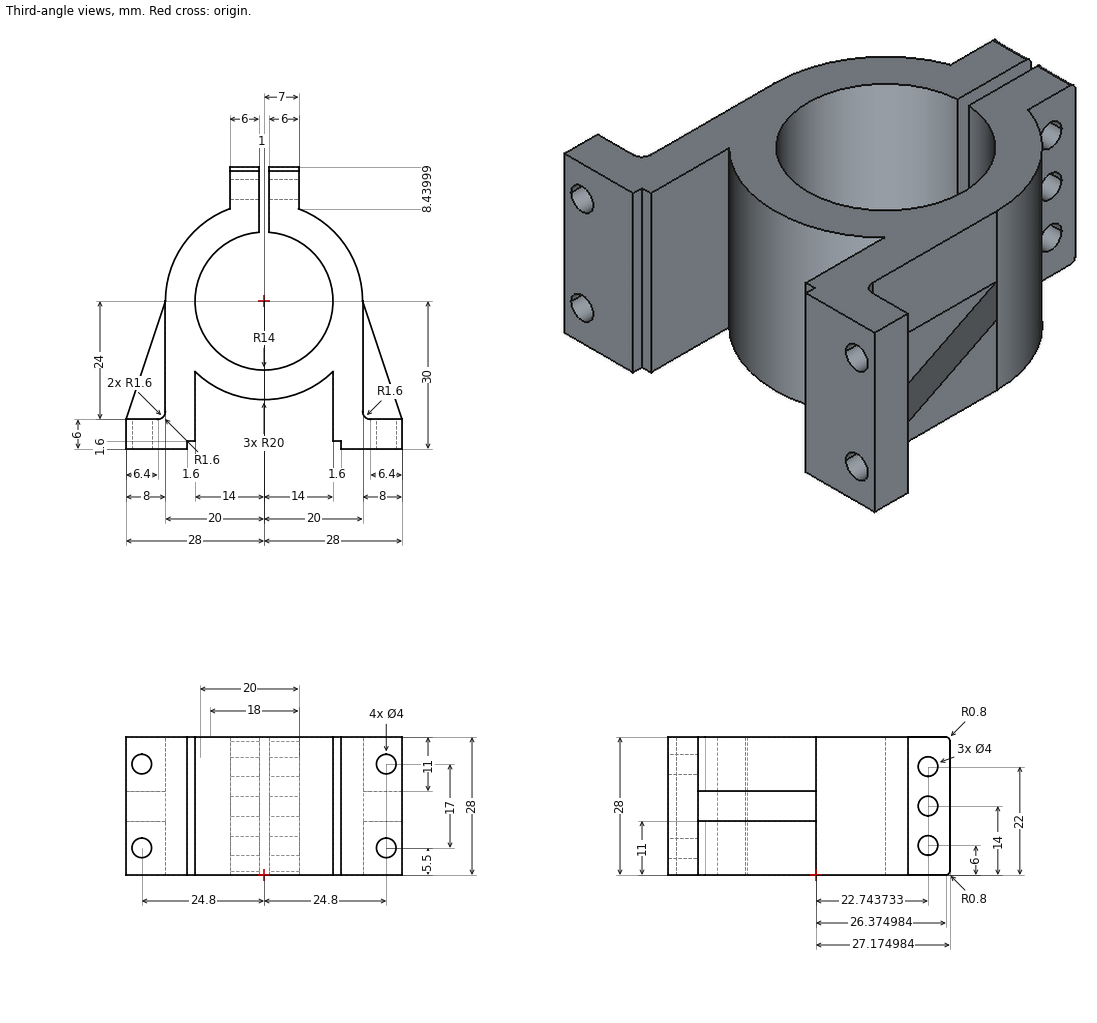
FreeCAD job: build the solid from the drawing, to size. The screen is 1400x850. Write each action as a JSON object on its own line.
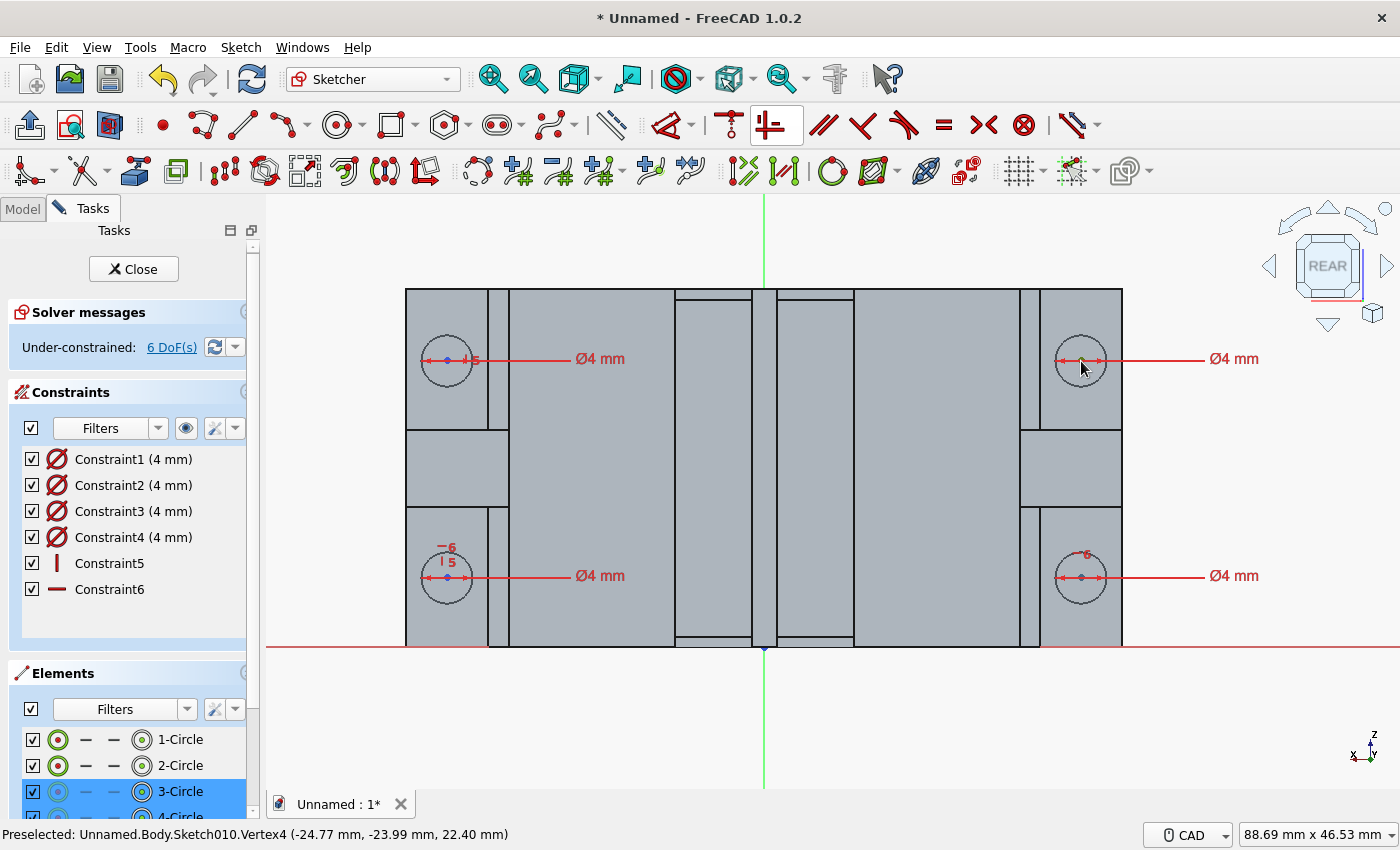
{"action": "key", "text": "v"}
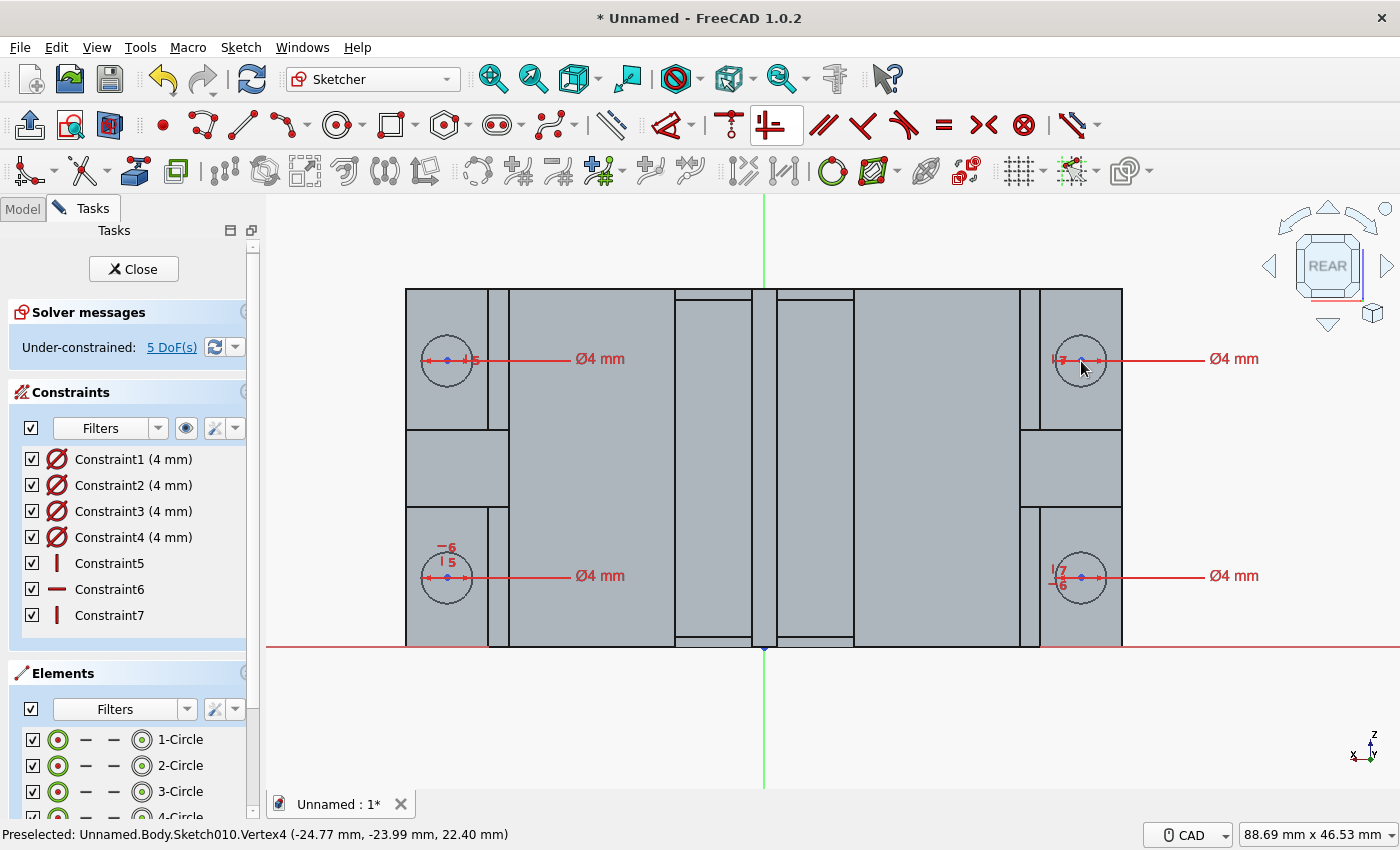
{"action": "left_click", "coordinate": [447, 361]}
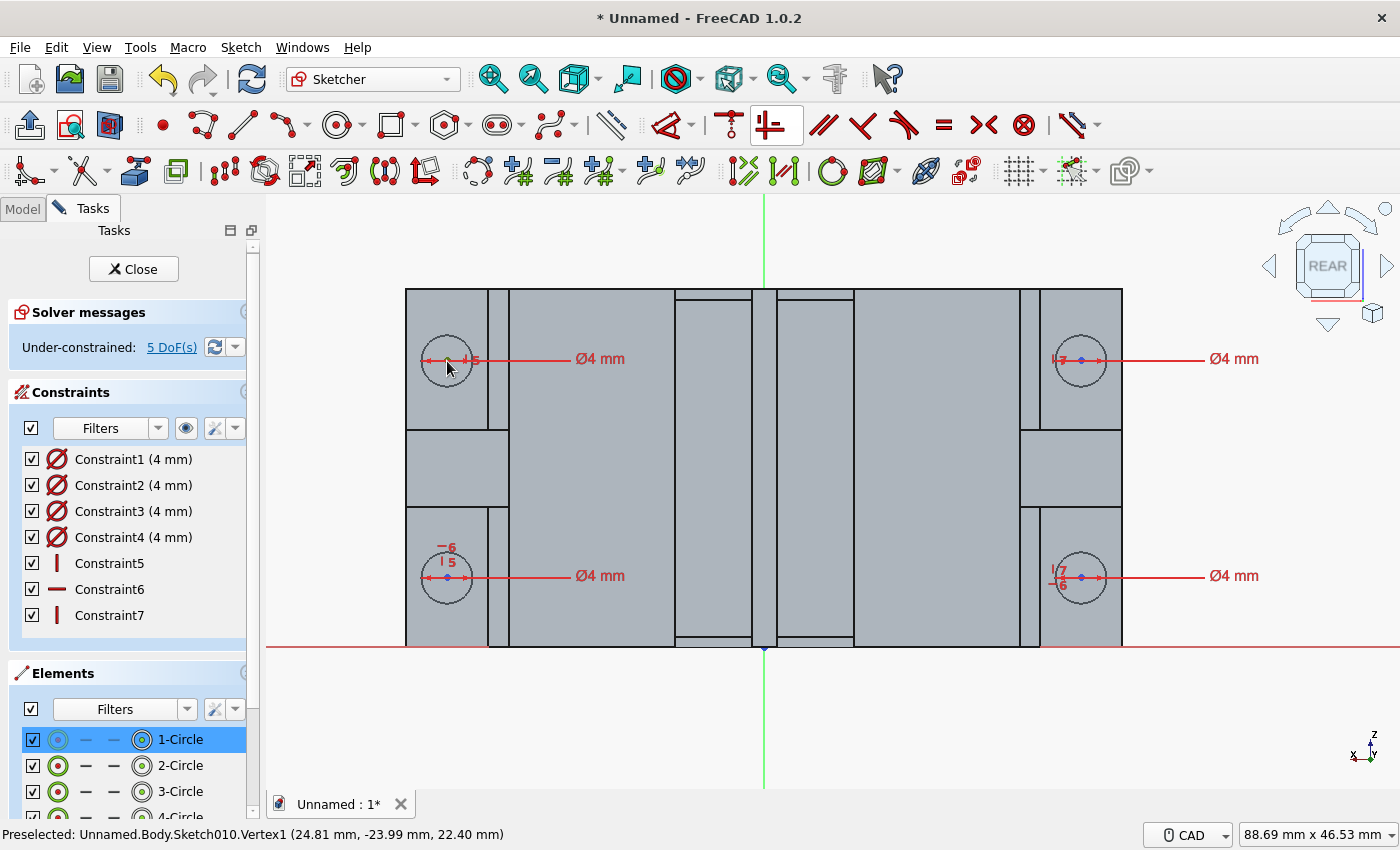
{"action": "left_click", "coordinate": [1081, 361]}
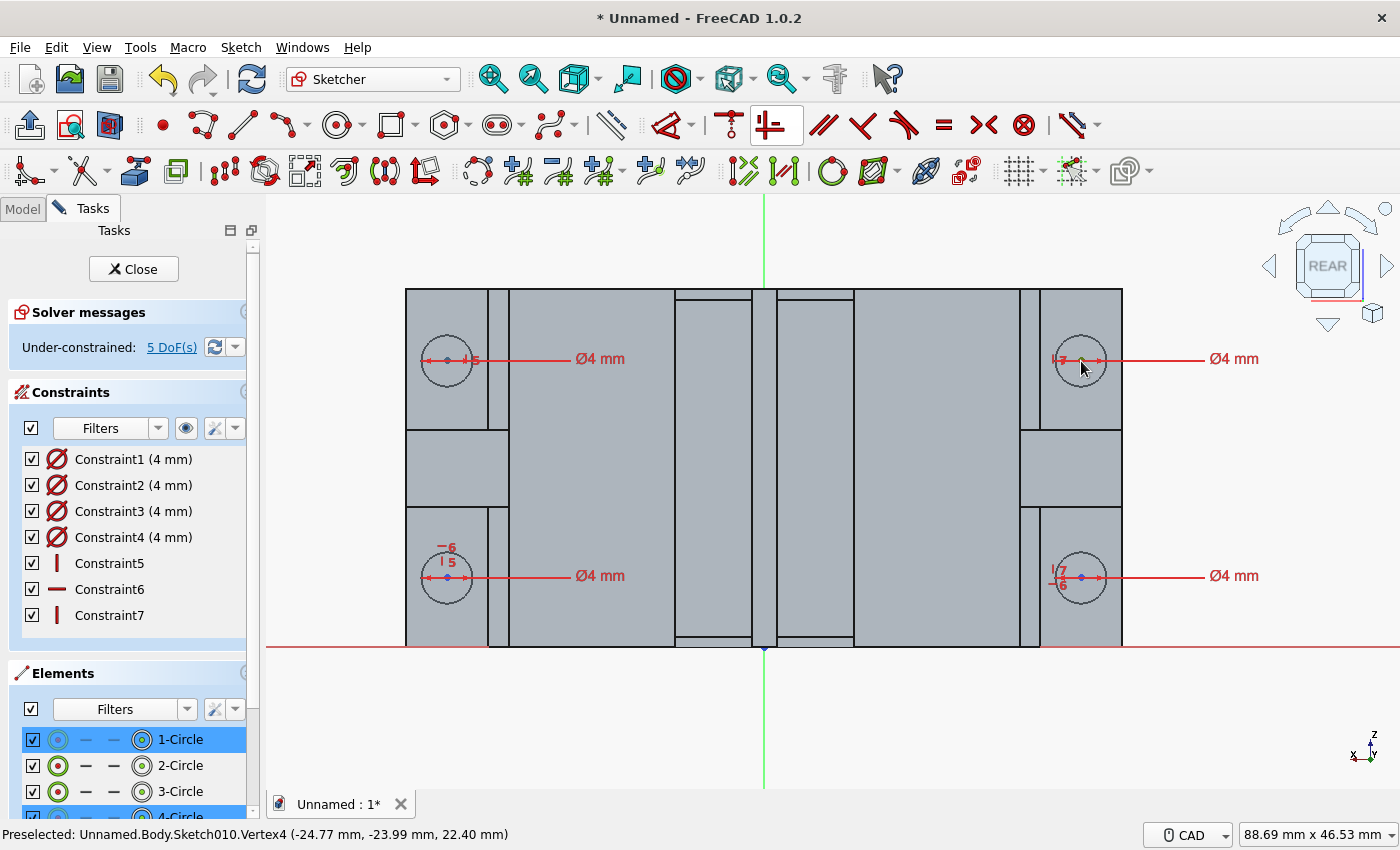
{"action": "left_click", "coordinate": [798, 126]}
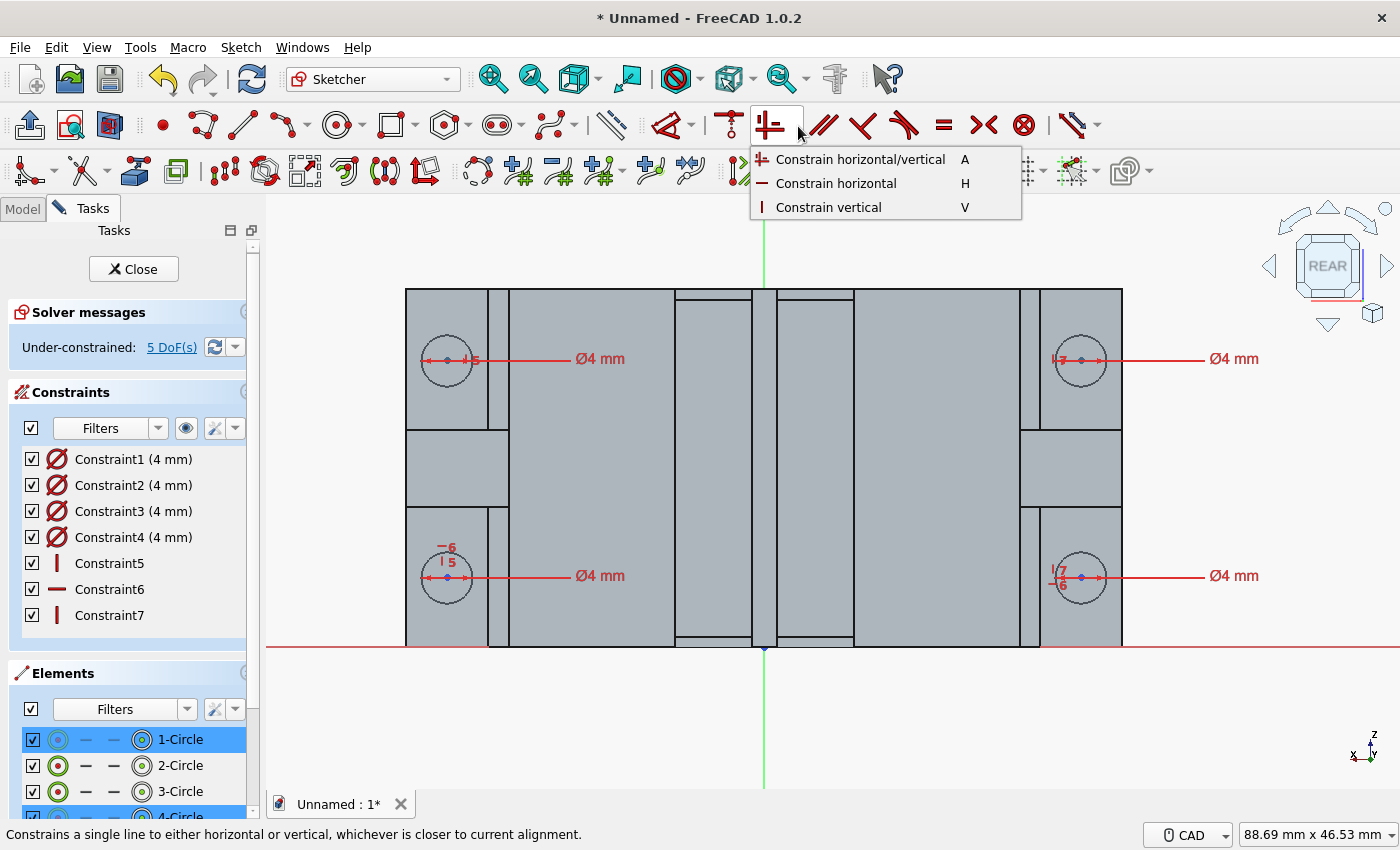
{"action": "left_click", "coordinate": [886, 183]}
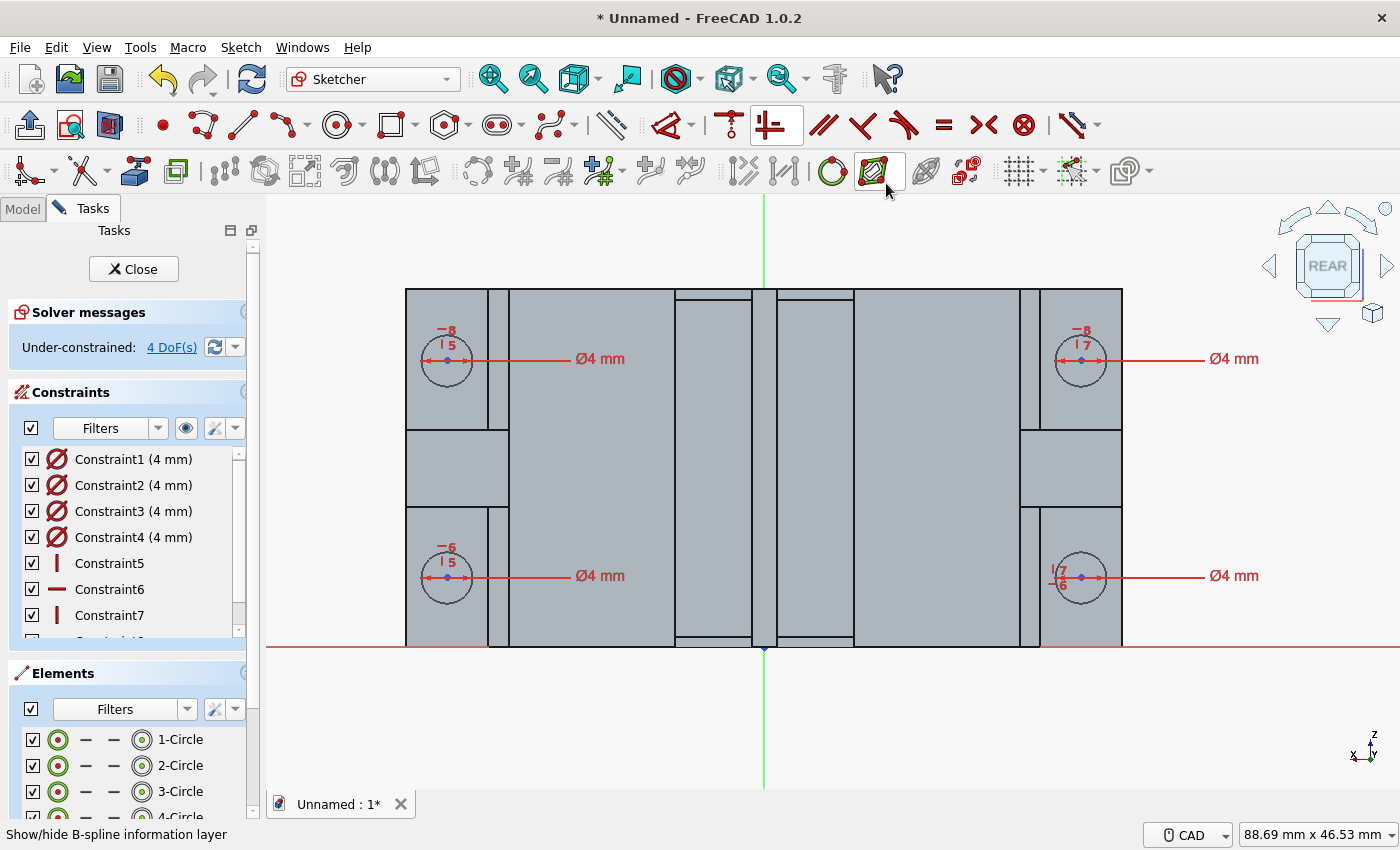
{"action": "left_click", "coordinate": [666, 126]}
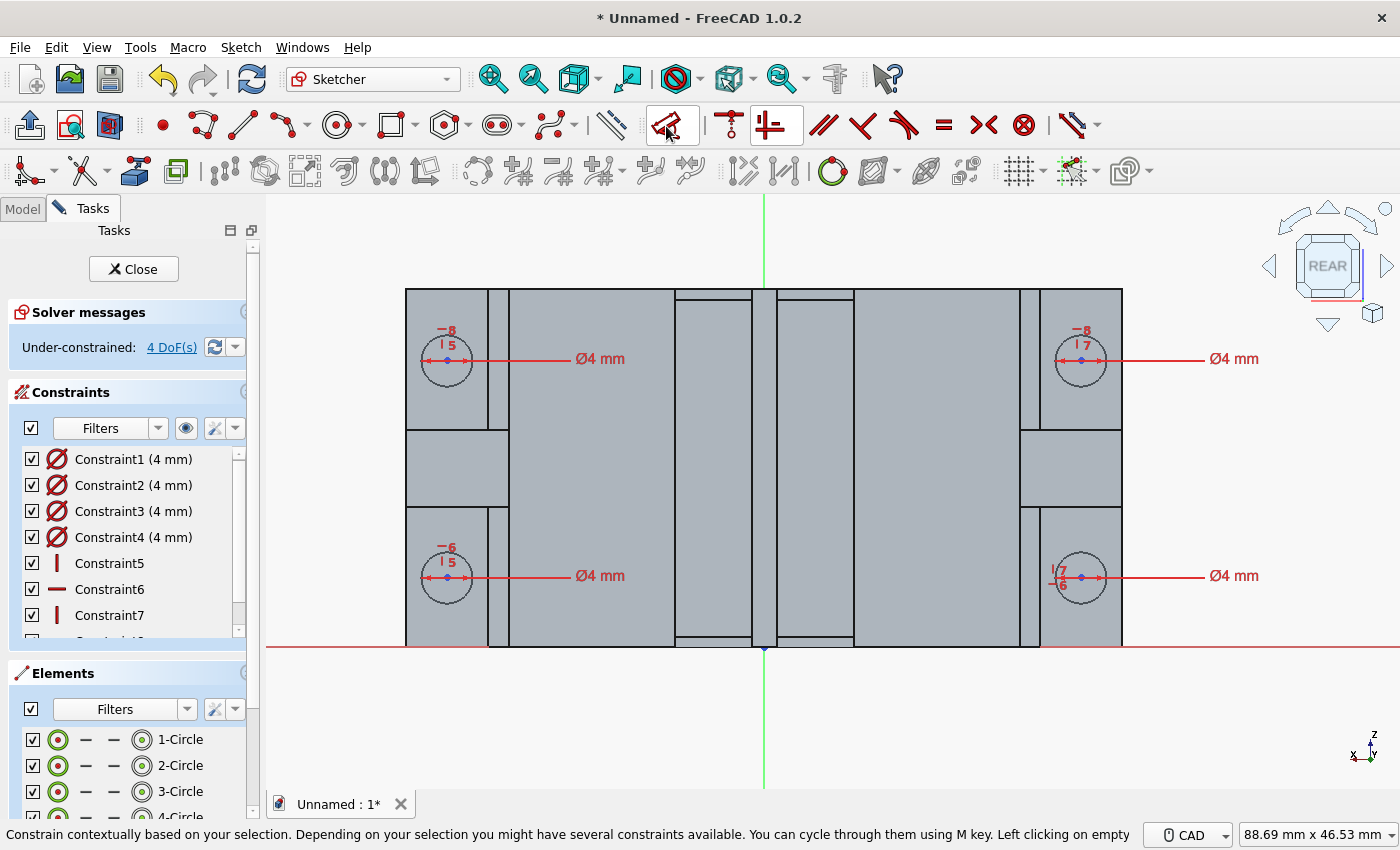
{"action": "left_click", "coordinate": [447, 578]}
{"action": "left_click", "coordinate": [413, 613]}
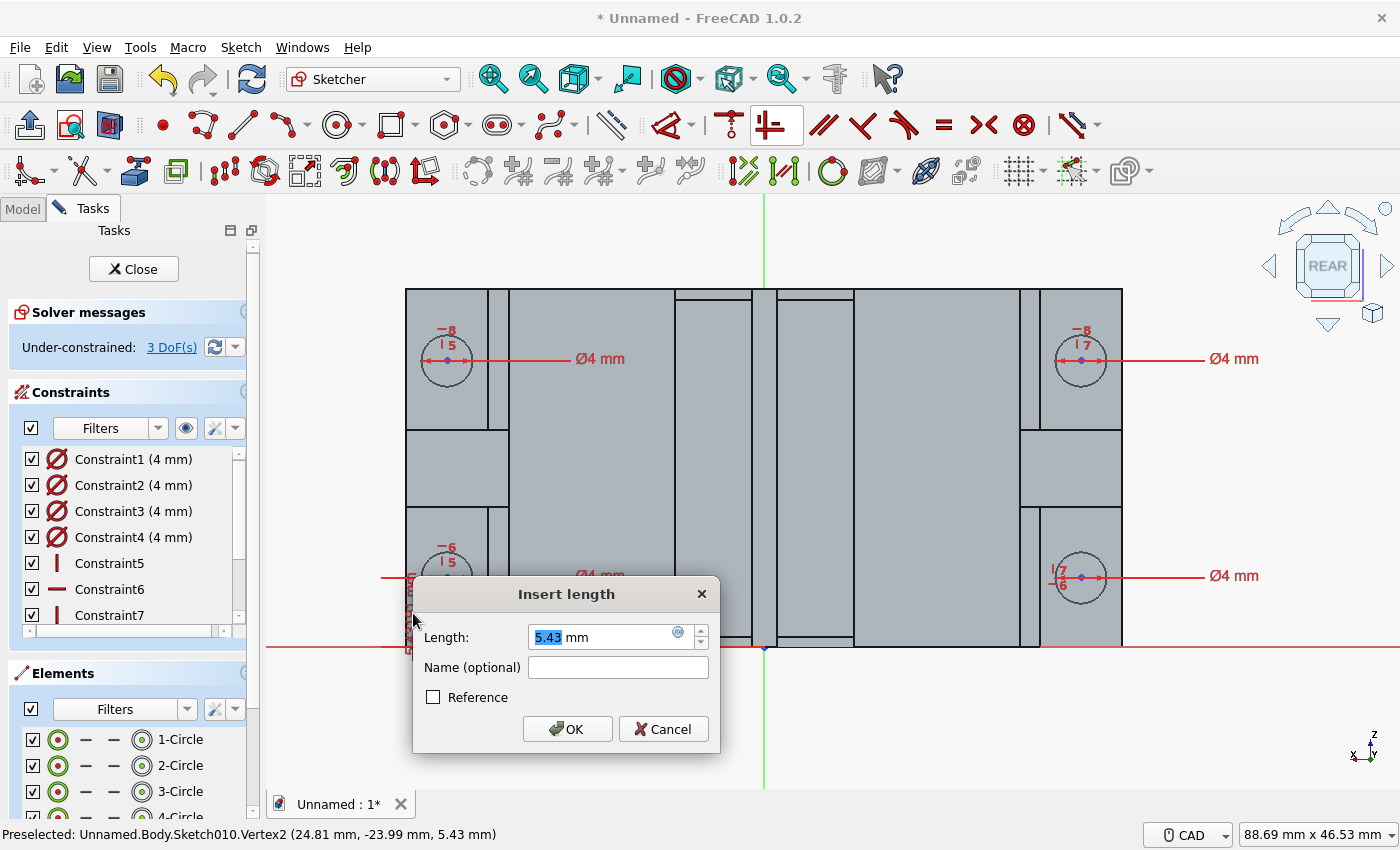
{"action": "type", "text": "5.5"}
{"action": "key", "text": "Return"}